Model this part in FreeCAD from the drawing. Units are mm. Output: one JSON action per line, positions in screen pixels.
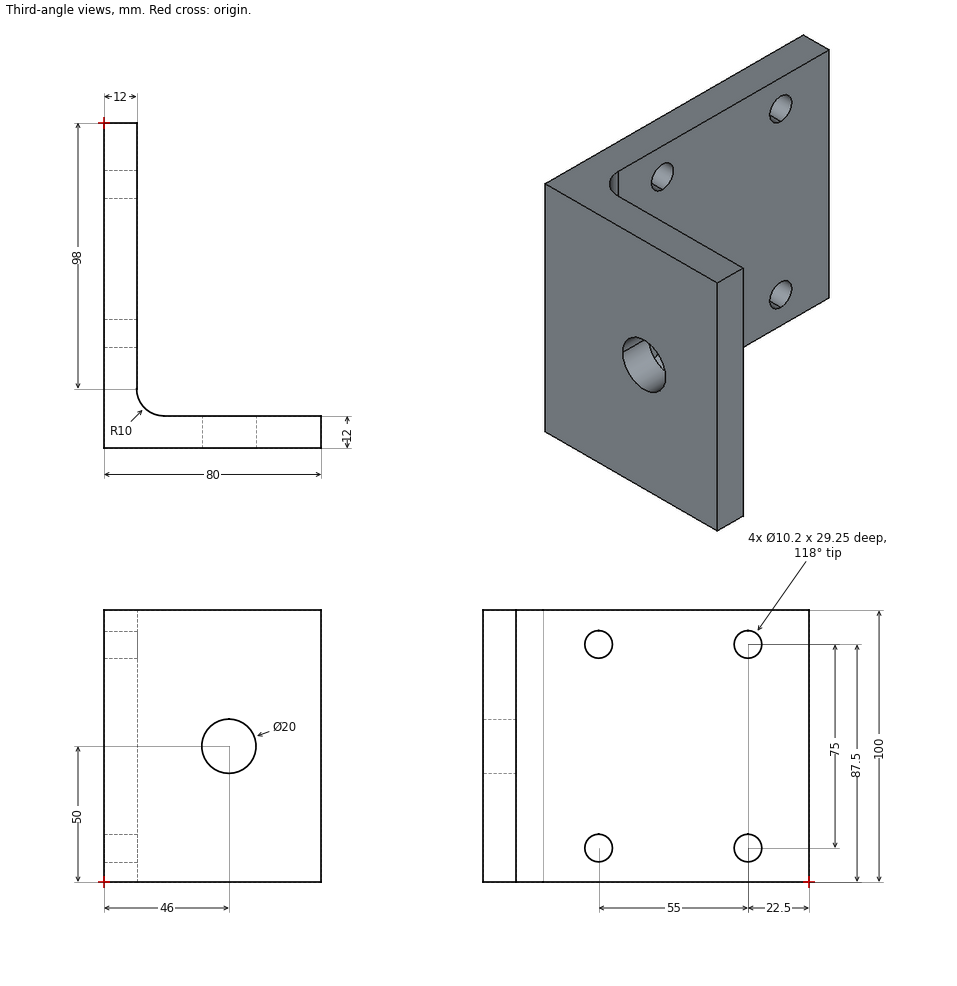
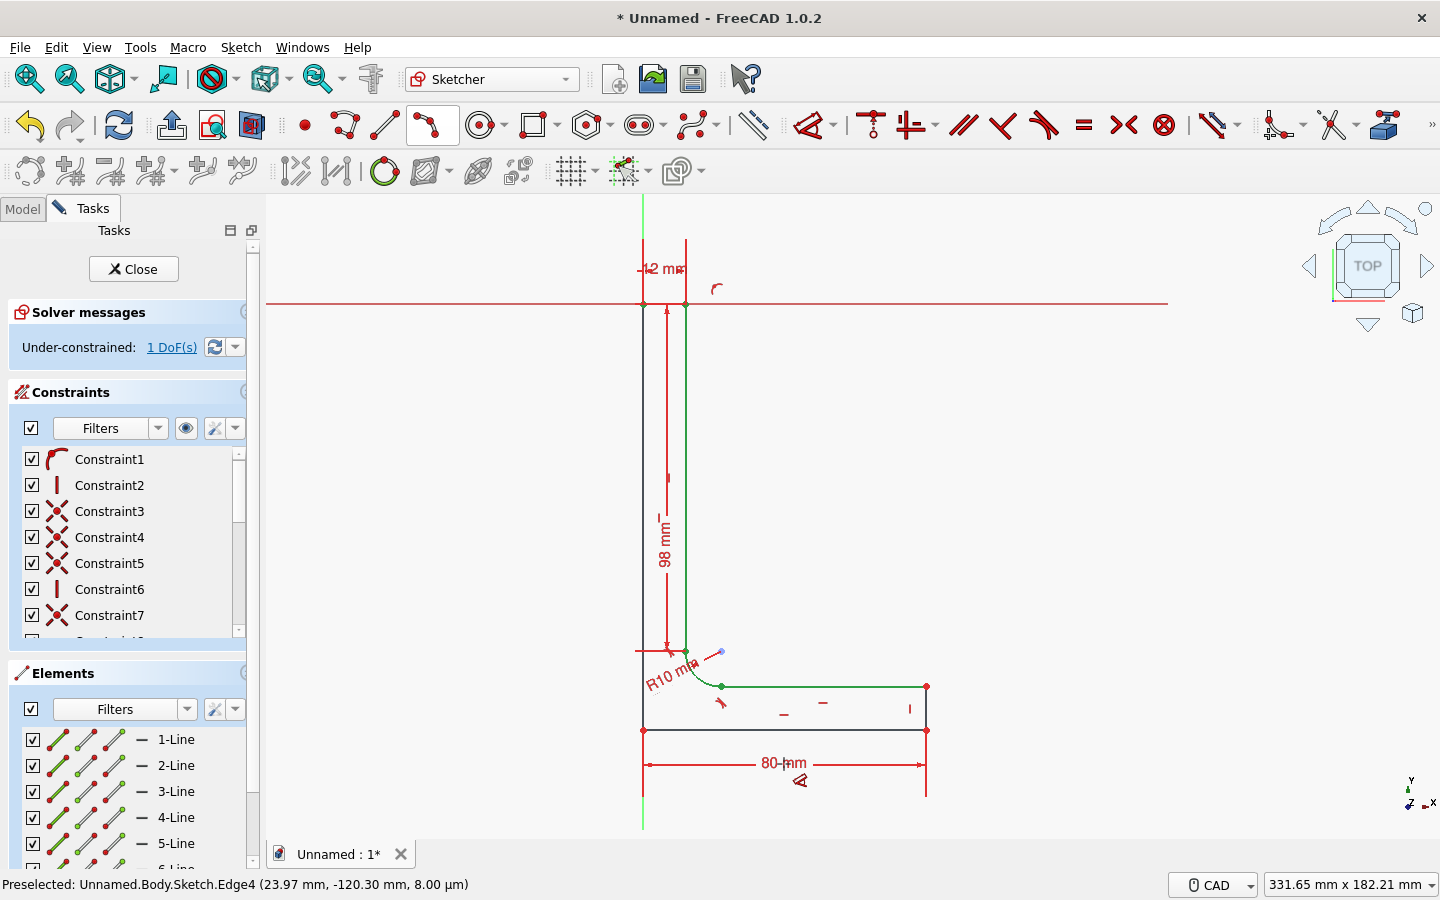
{"action": "left_click", "coordinate": [926, 717]}
{"action": "left_click", "coordinate": [960, 708]}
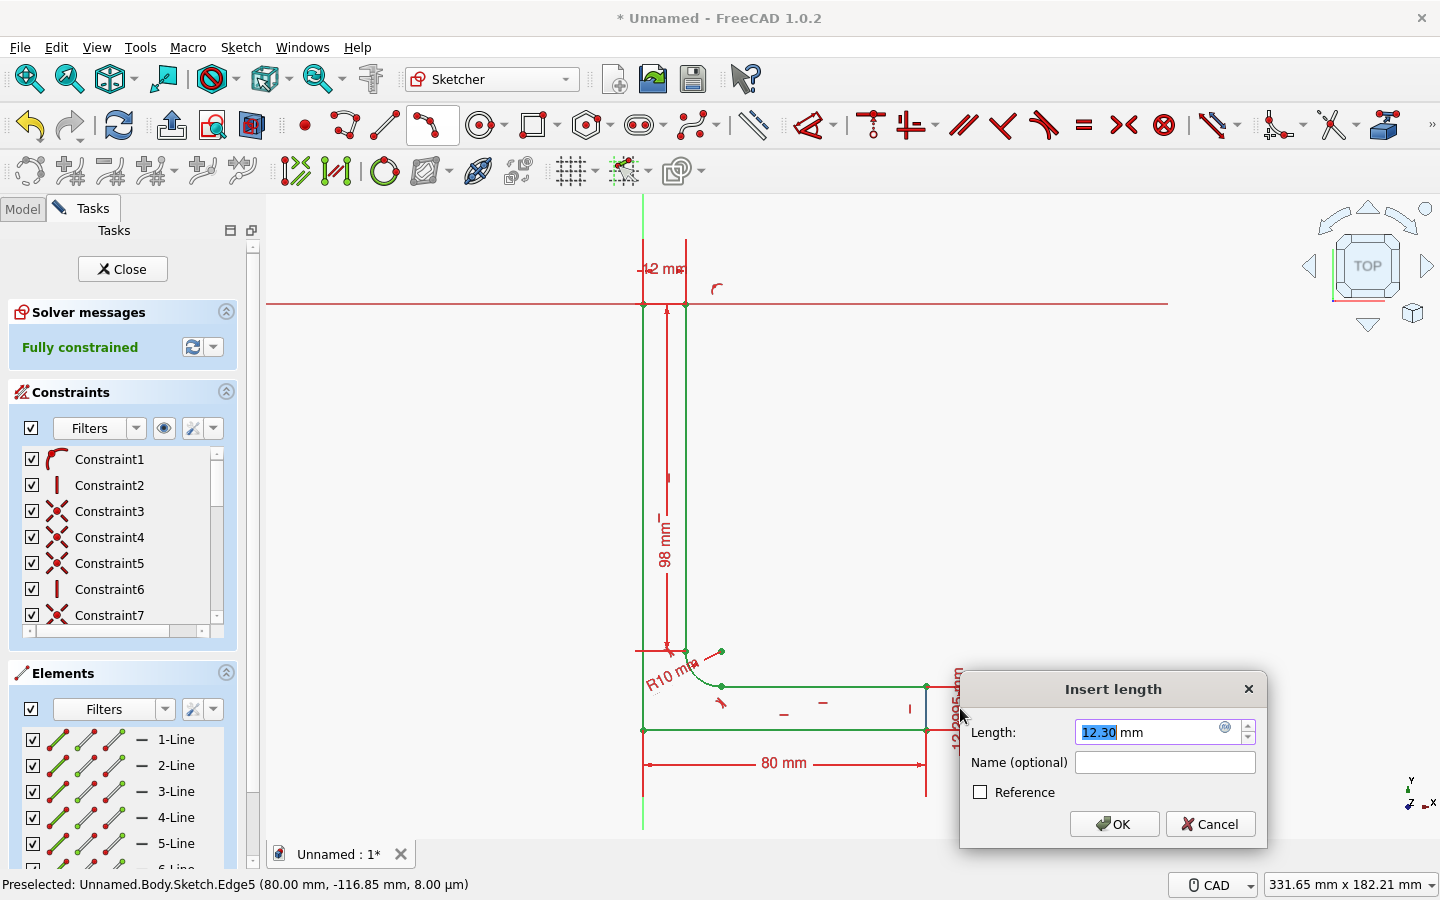
{"action": "type", "text": "12"}
{"action": "key", "text": "Return"}
{"action": "key", "text": "Escape"}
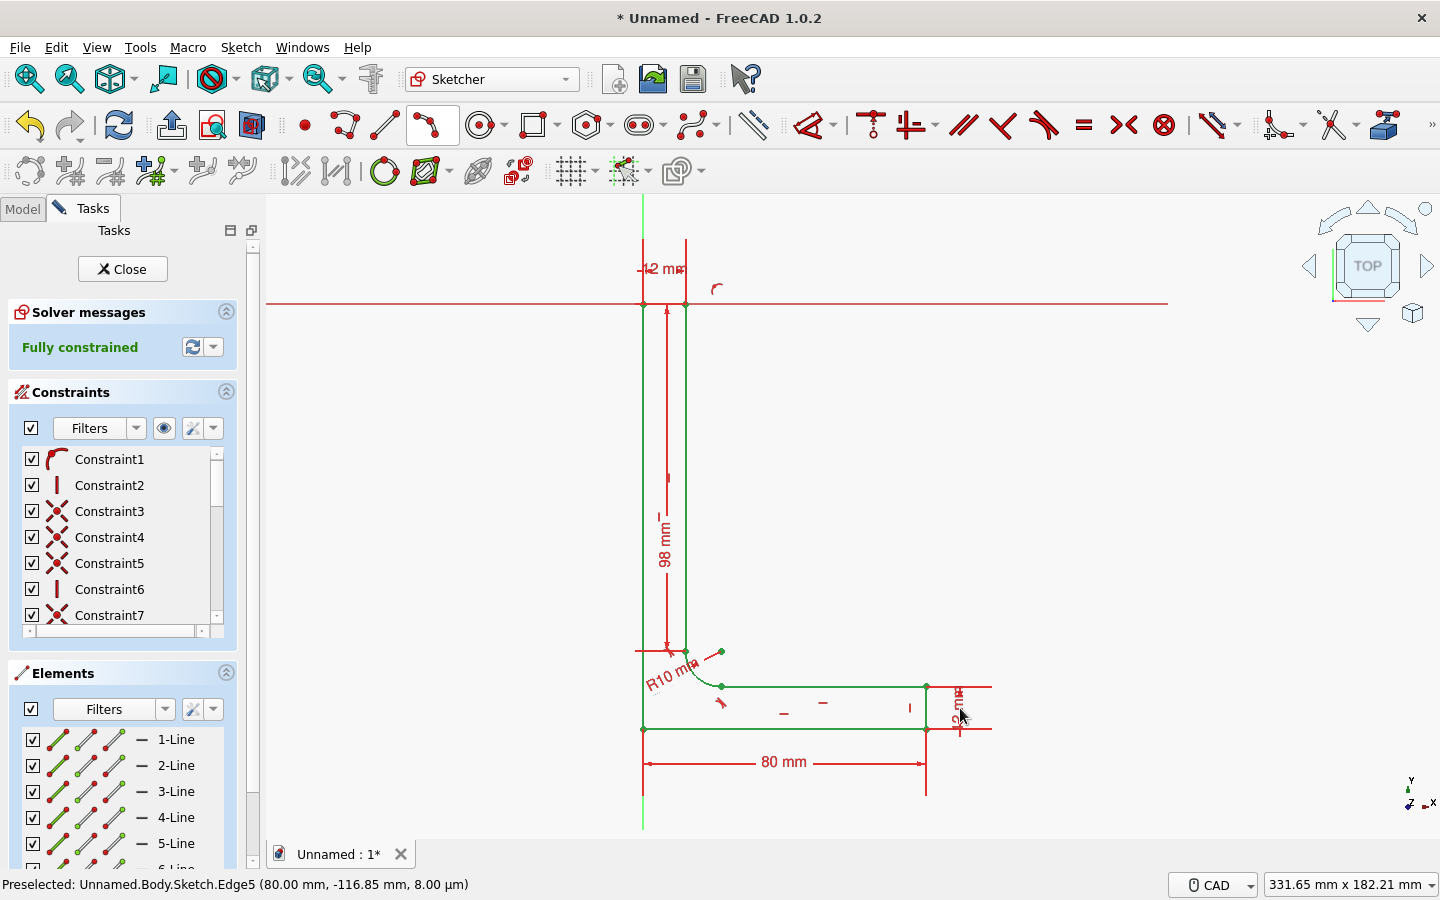
{"action": "left_click", "coordinate": [123, 269]}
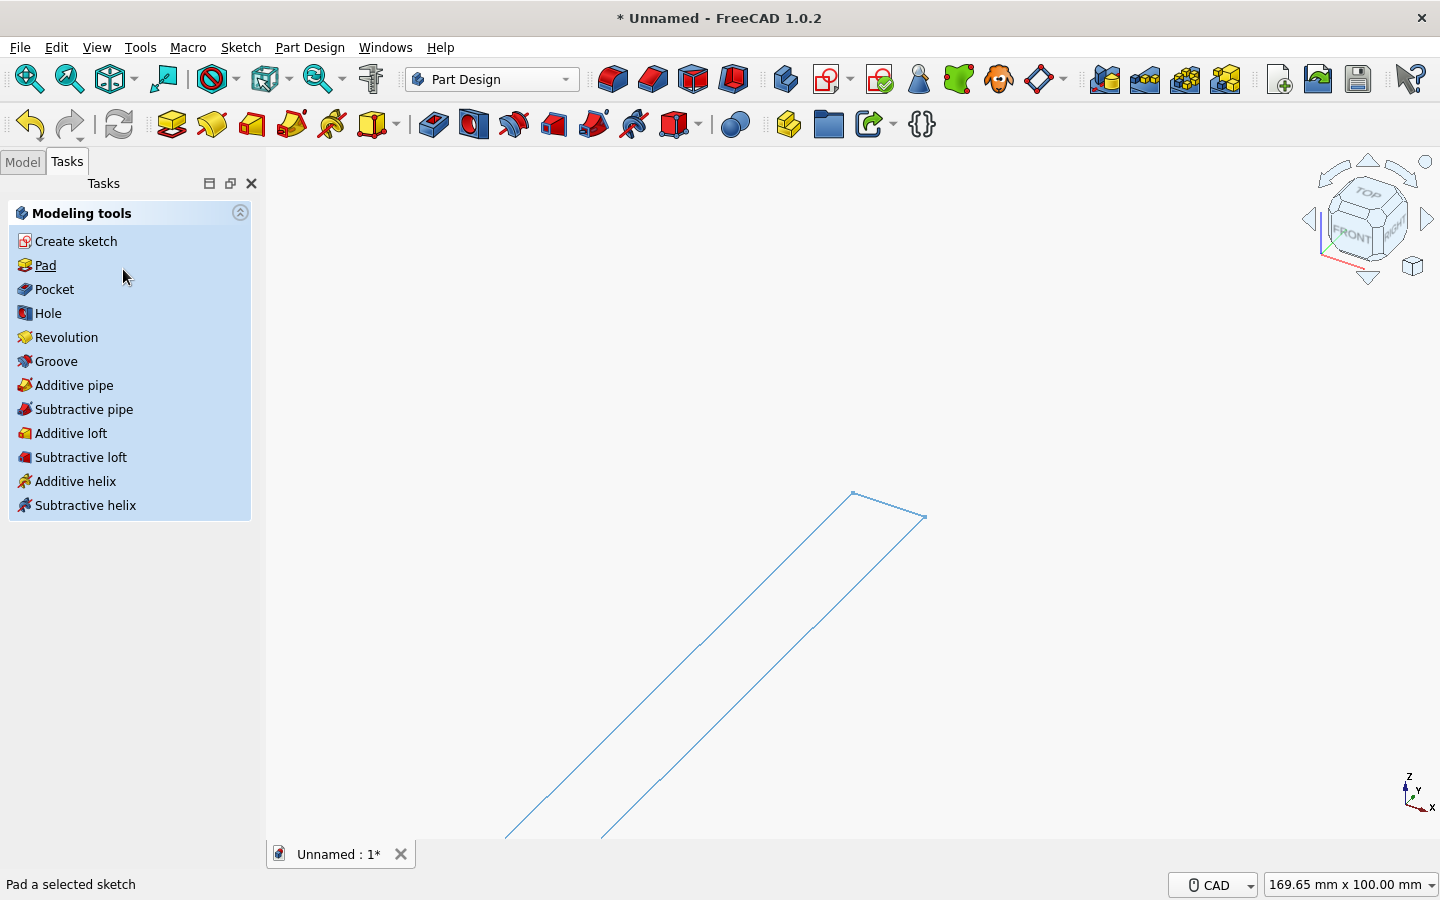
{"action": "left_click", "coordinate": [172, 124]}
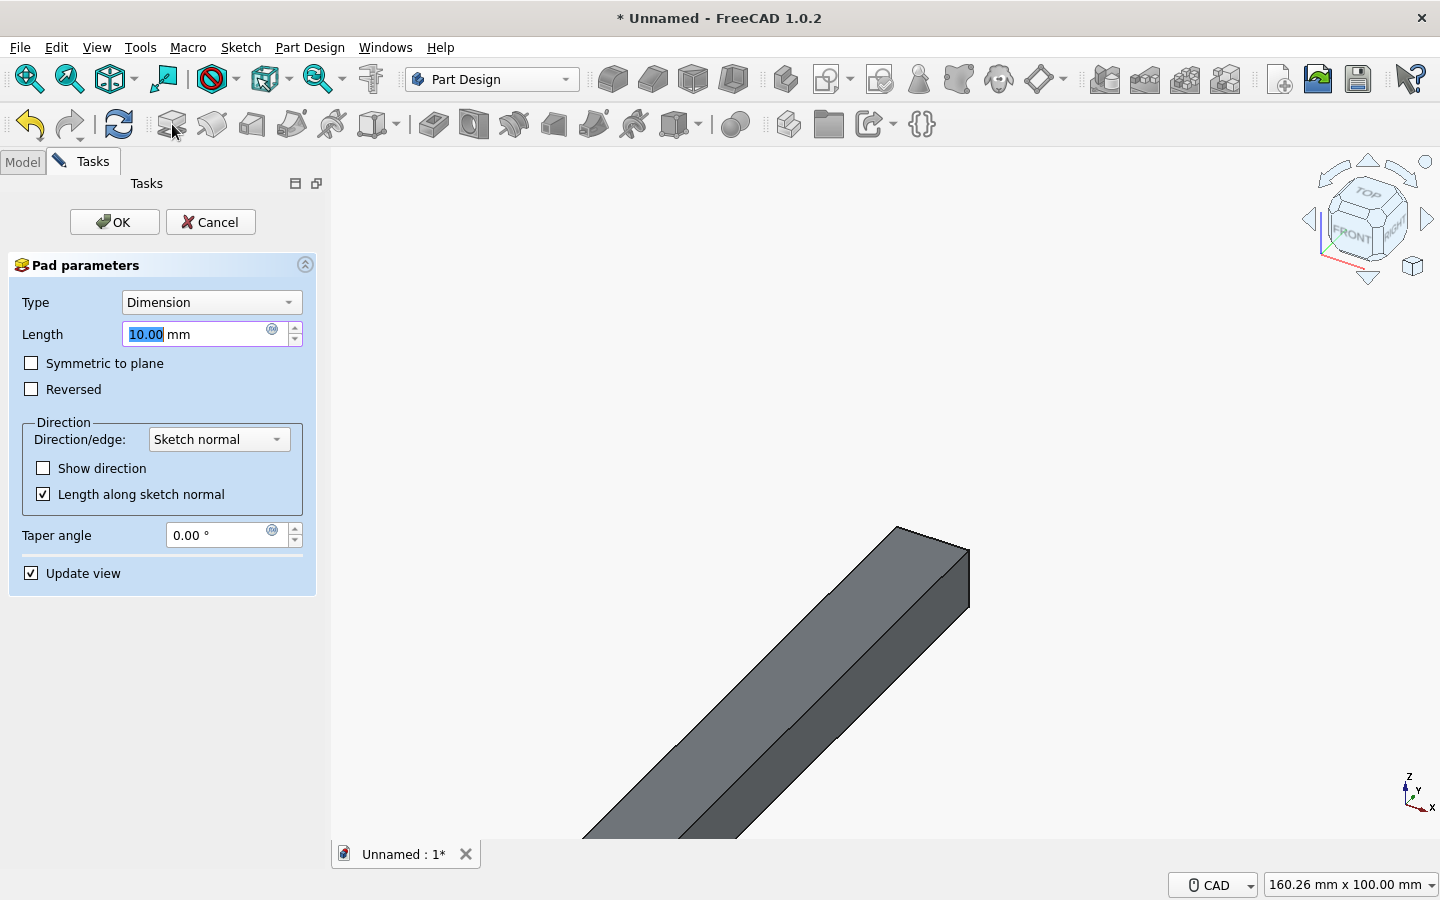
{"action": "type", "text": "100"}
{"action": "key", "text": "Tab"}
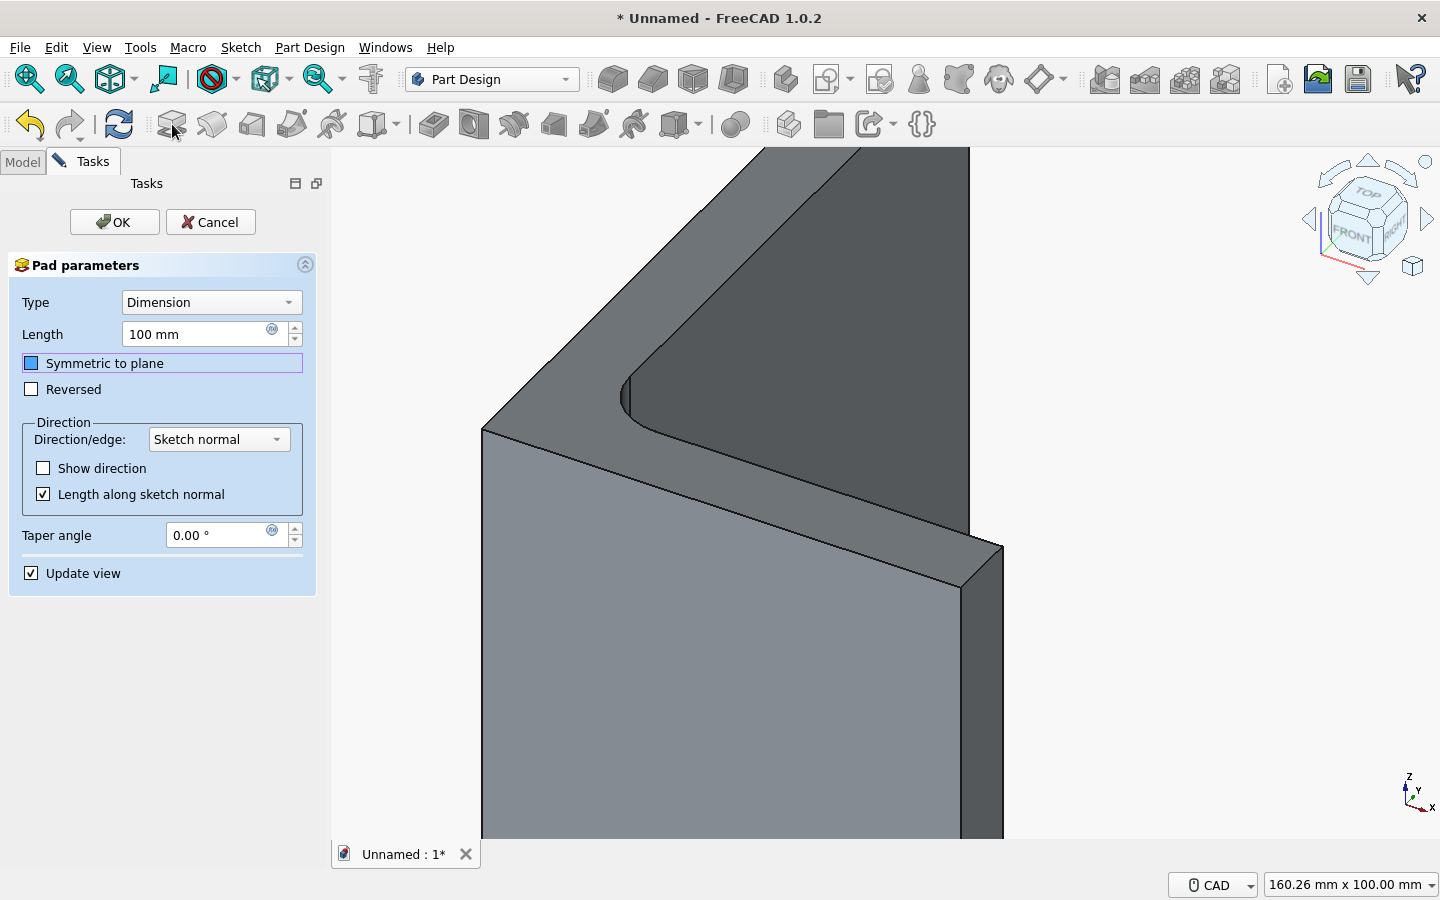
{"action": "left_click", "coordinate": [115, 222]}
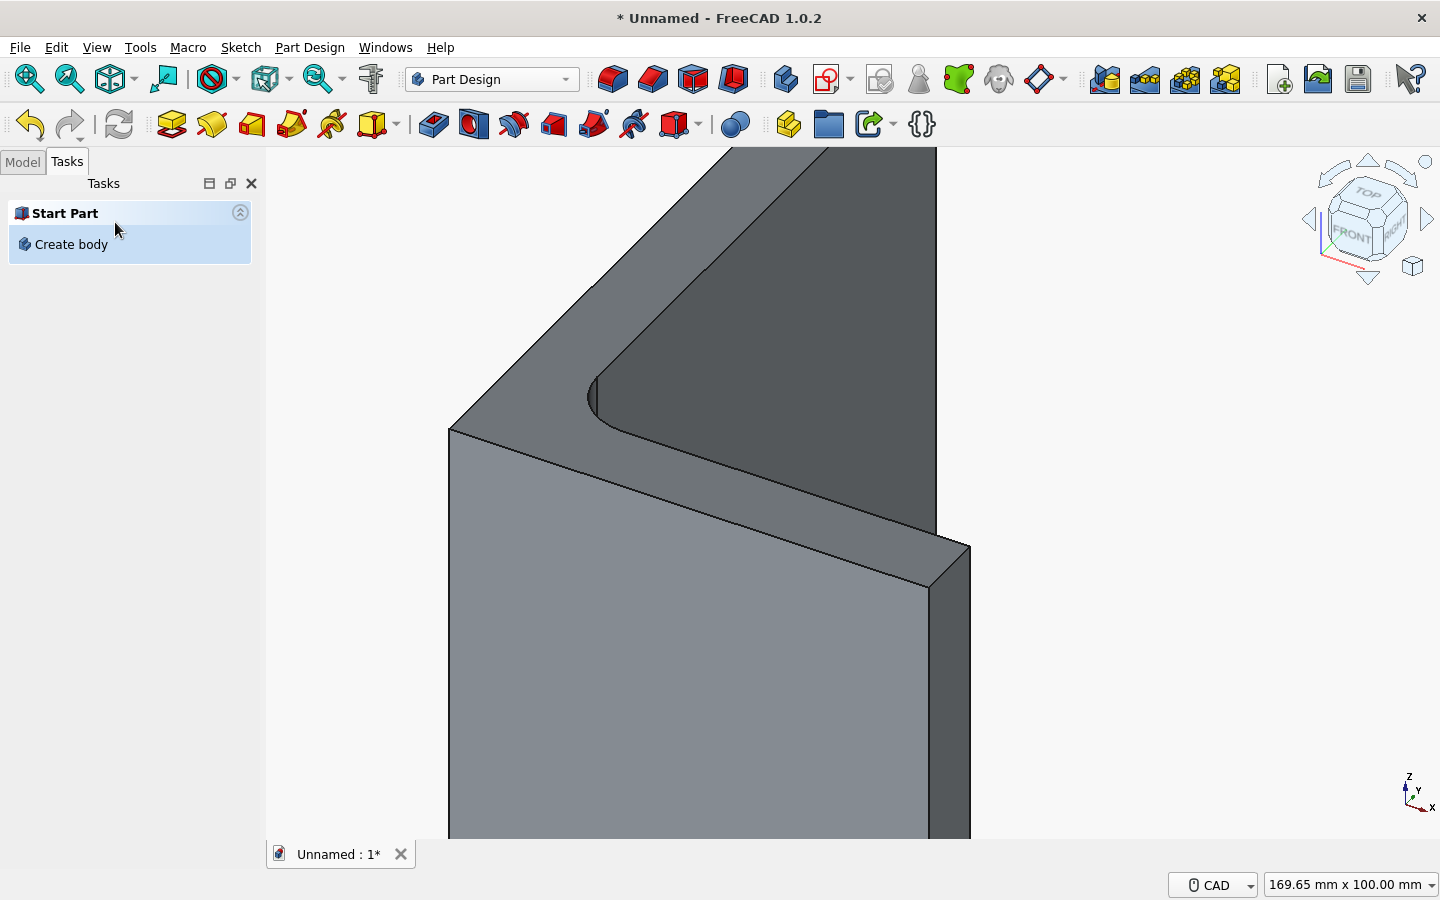
{"action": "left_click", "coordinate": [30, 80]}